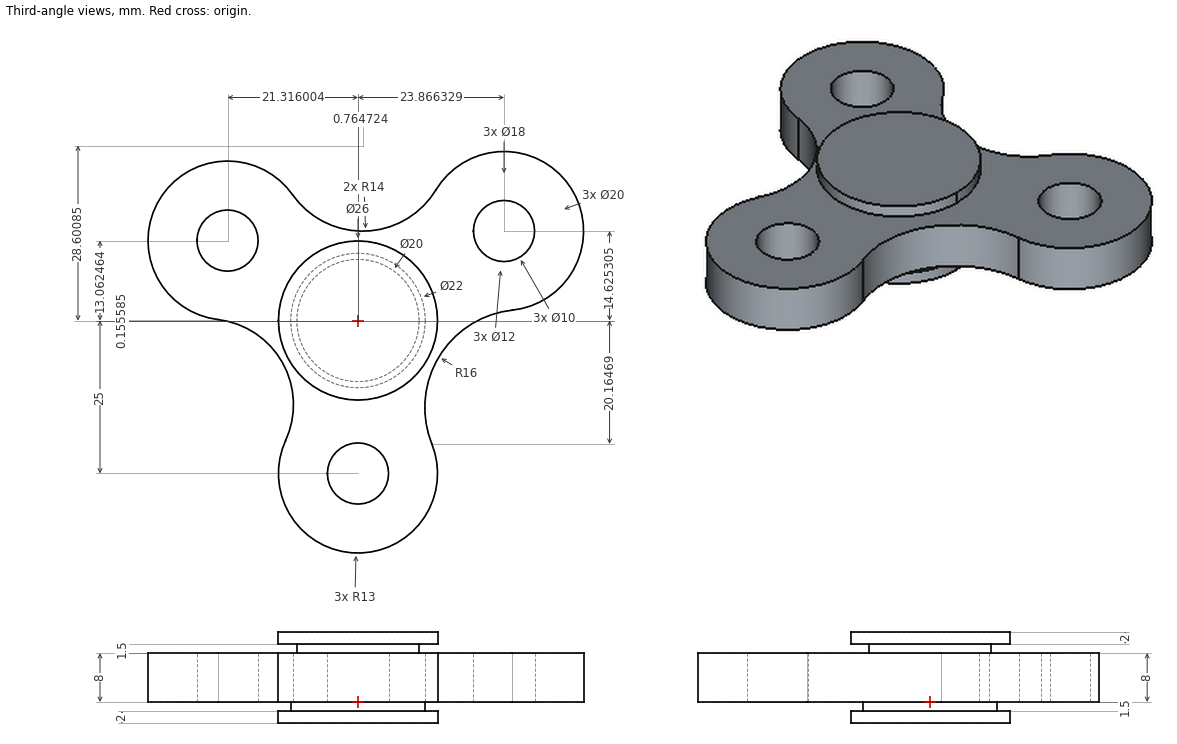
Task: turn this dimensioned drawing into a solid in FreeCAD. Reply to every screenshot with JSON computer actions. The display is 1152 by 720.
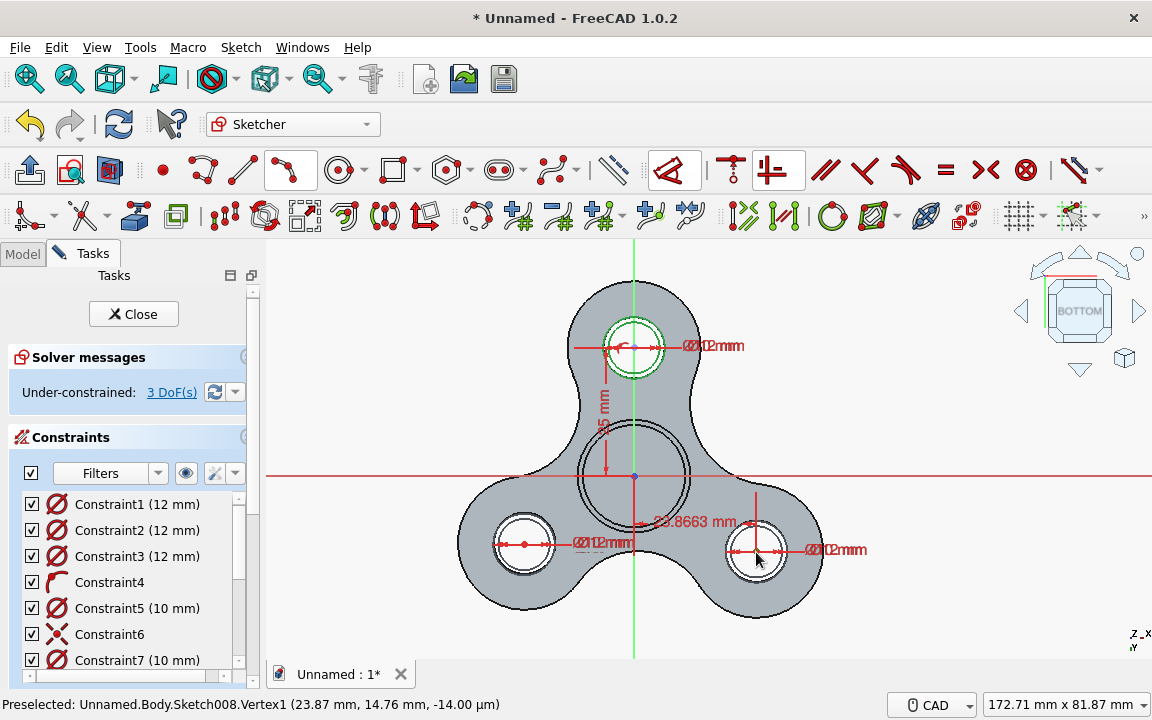
{"action": "left_click", "coordinate": [696, 170]}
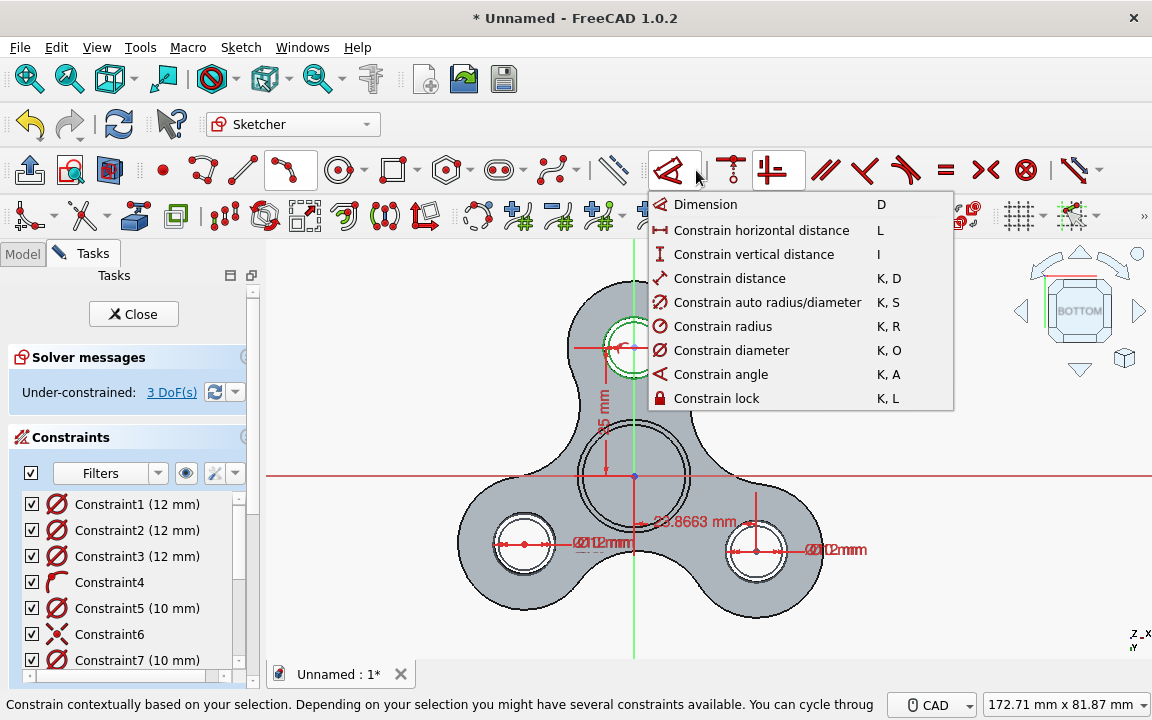
{"action": "left_click", "coordinate": [801, 254]}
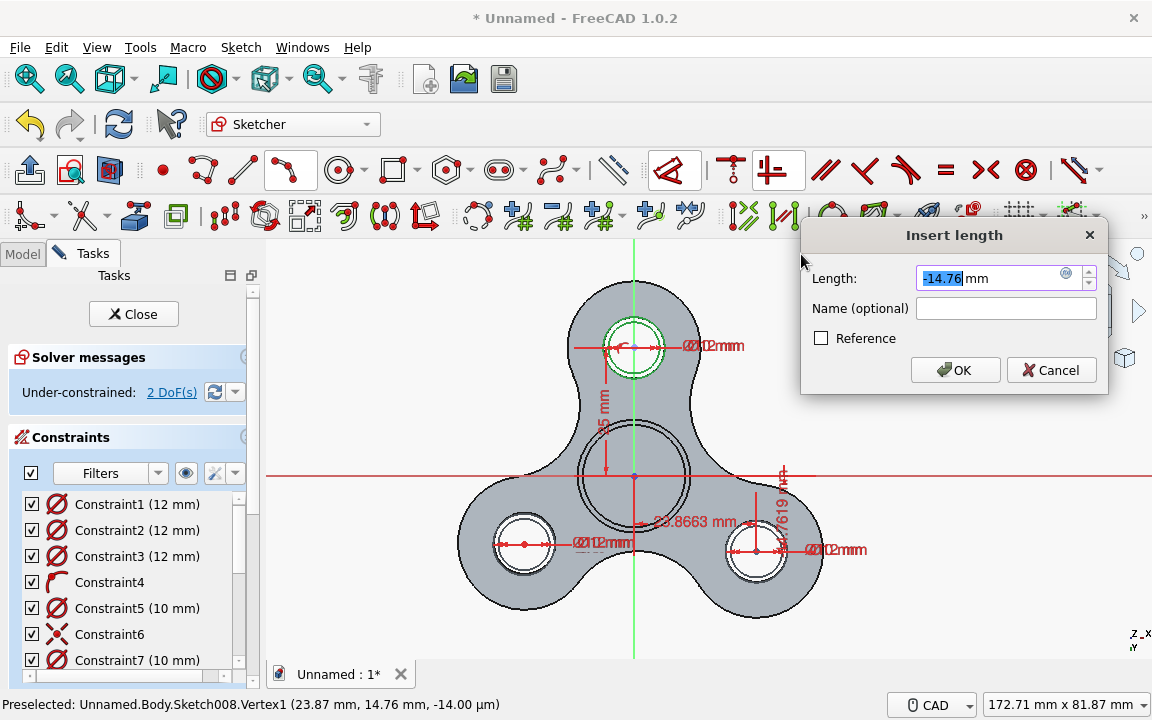
{"action": "type", "text": "-14.625305"}
{"action": "key", "text": "Return"}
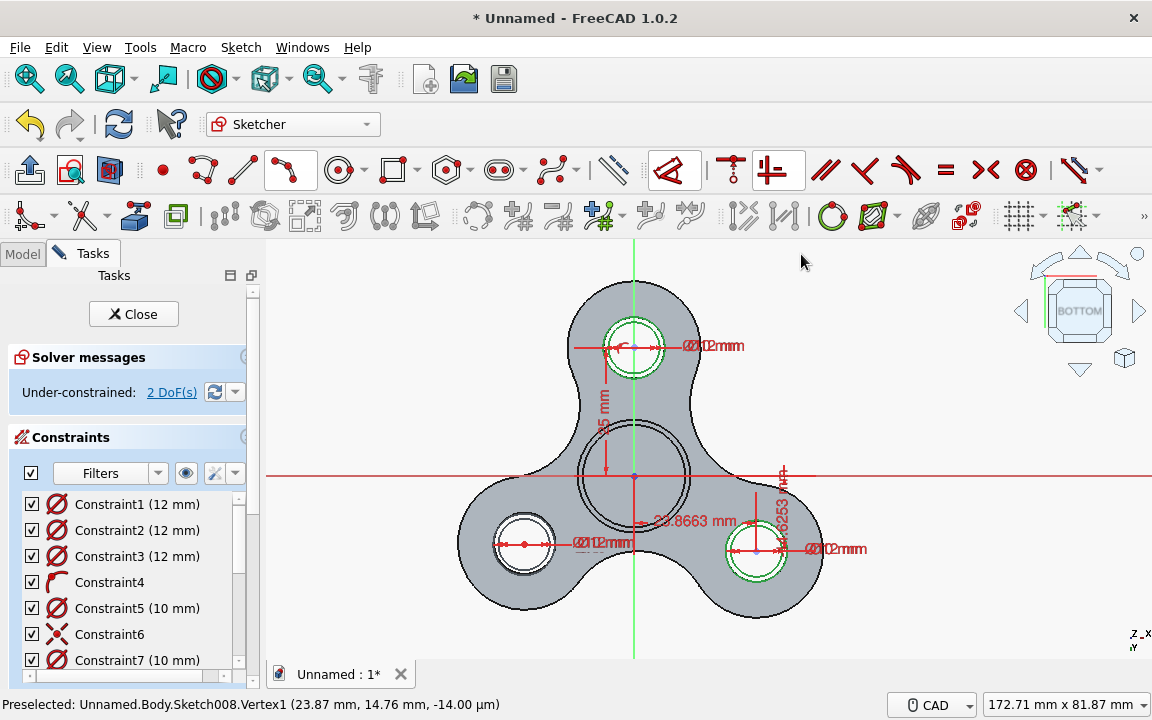
{"action": "left_click", "coordinate": [524, 545]}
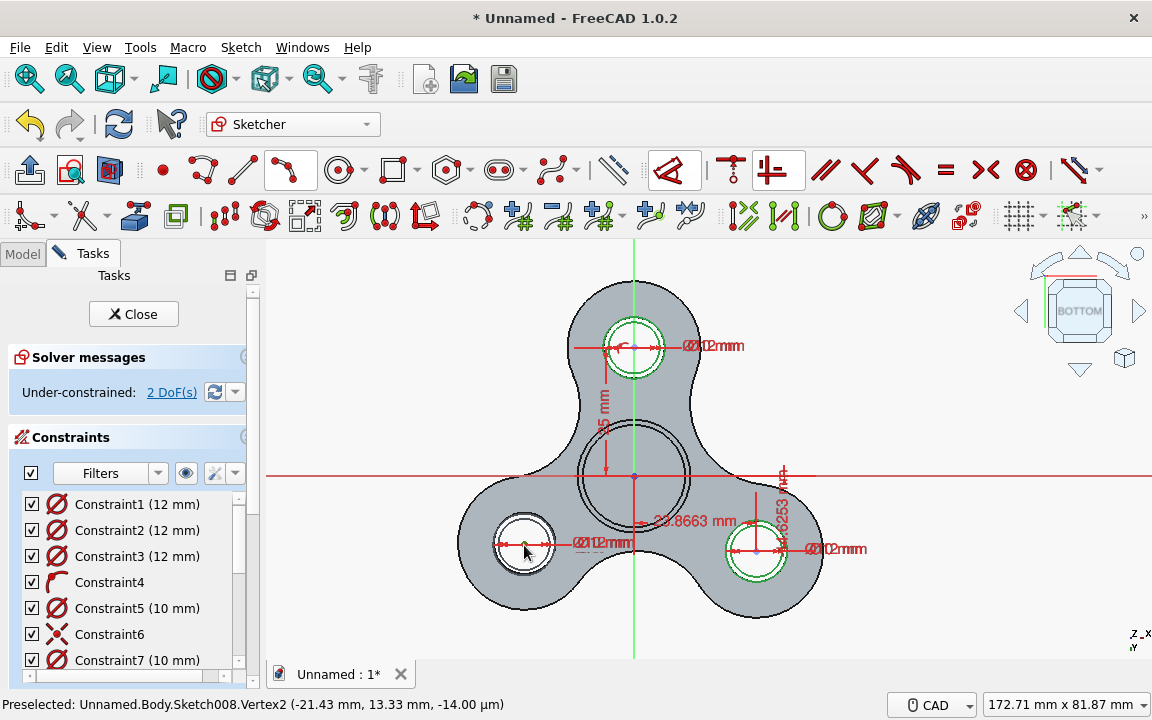
{"action": "left_click", "coordinate": [696, 170]}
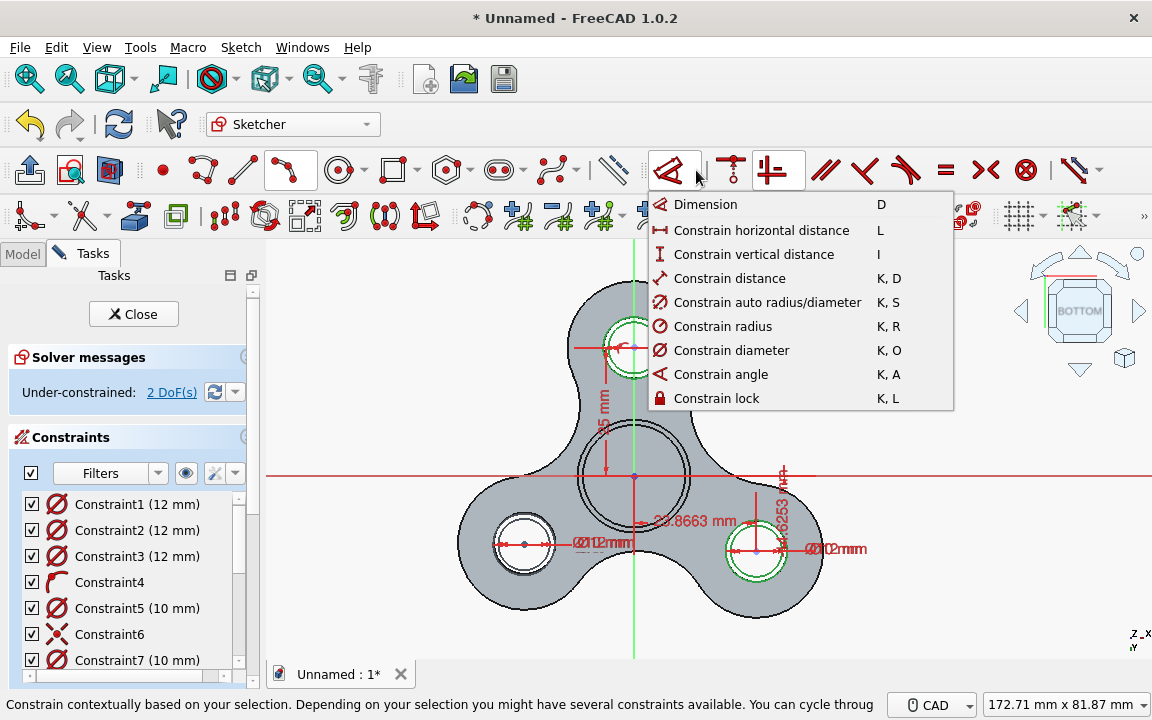
{"action": "left_click", "coordinate": [801, 230]}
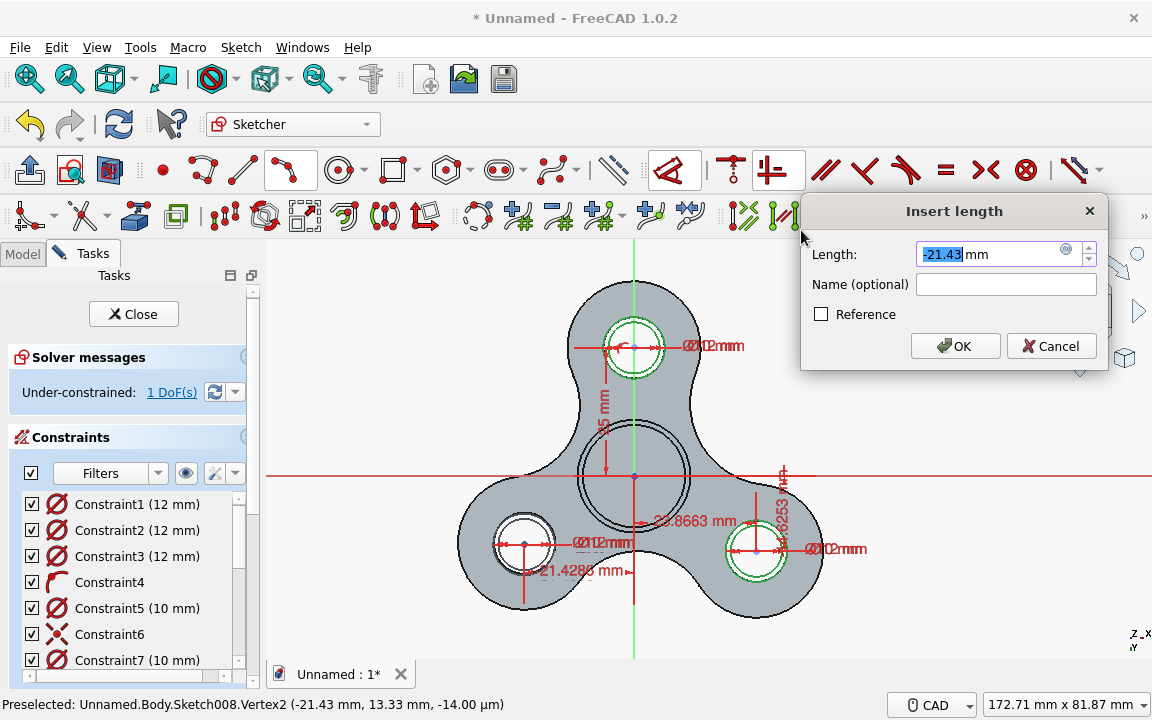
{"action": "type", "text": "-21.316004"}
{"action": "key", "text": "Return"}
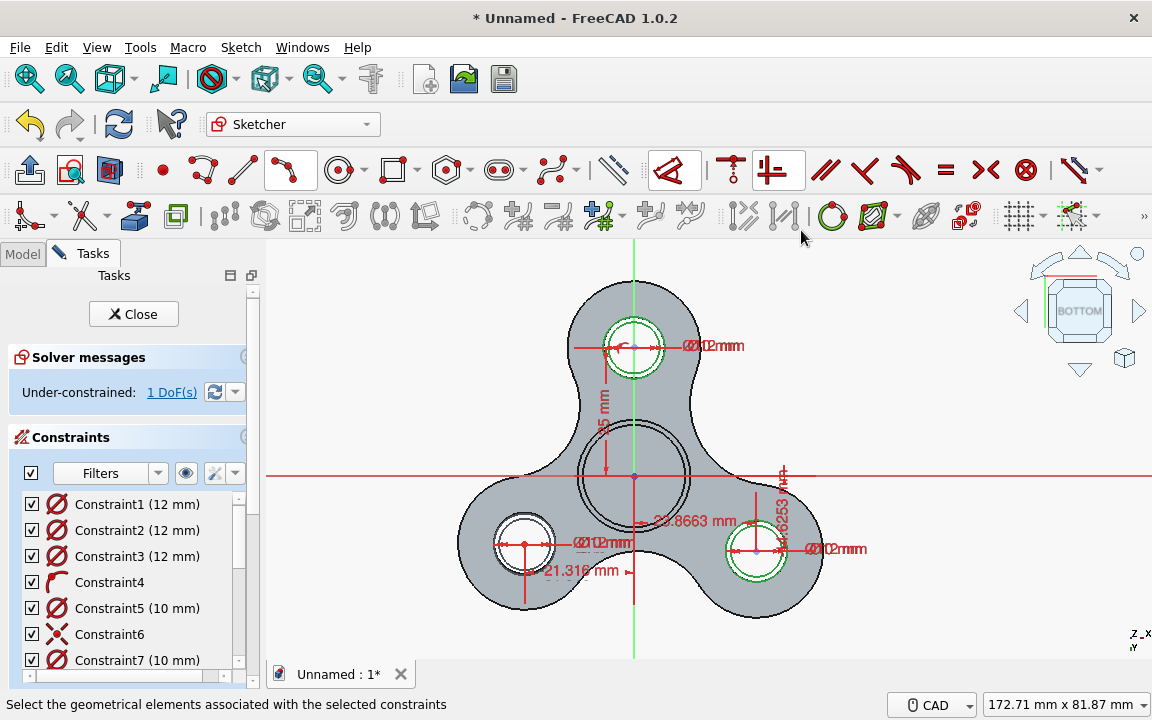
{"action": "left_click", "coordinate": [525, 545]}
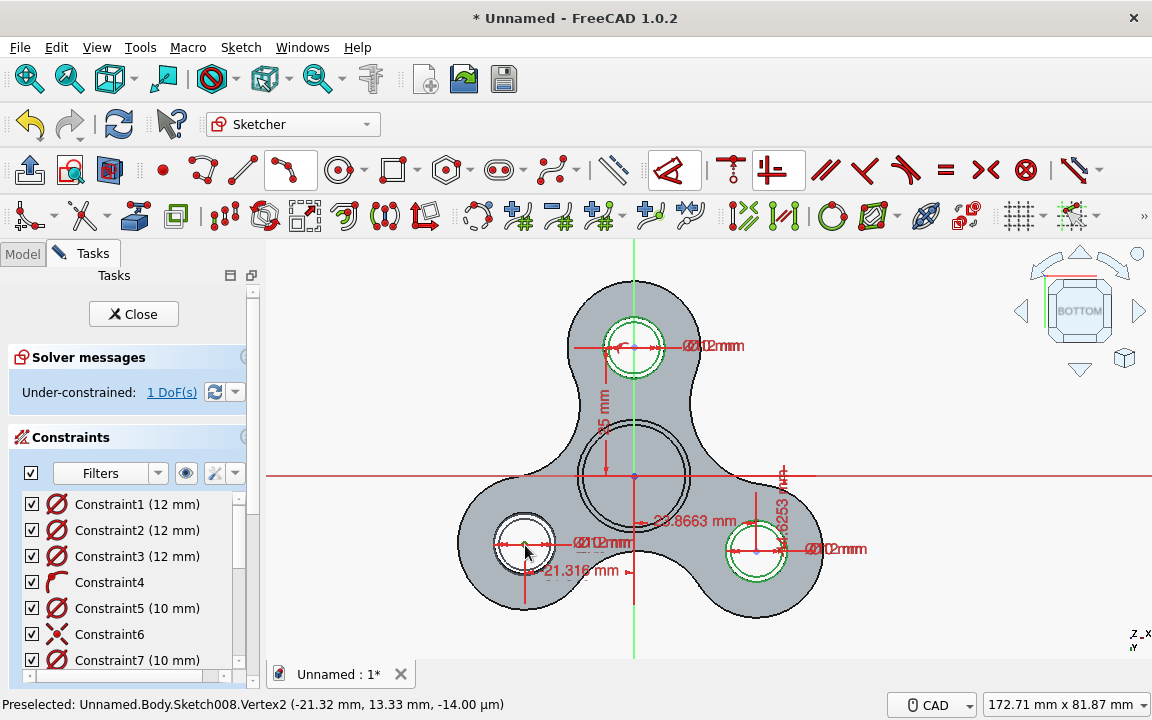
{"action": "key", "text": "i"}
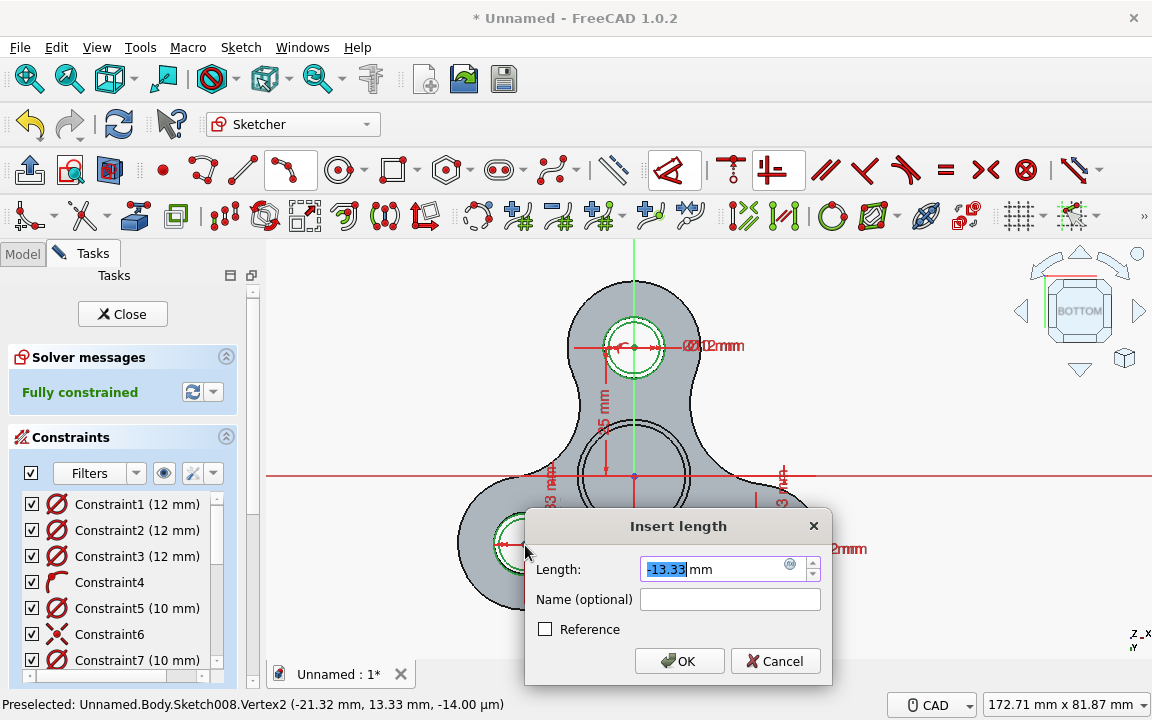
{"action": "type", "text": "-13.062464"}
{"action": "key", "text": "Return"}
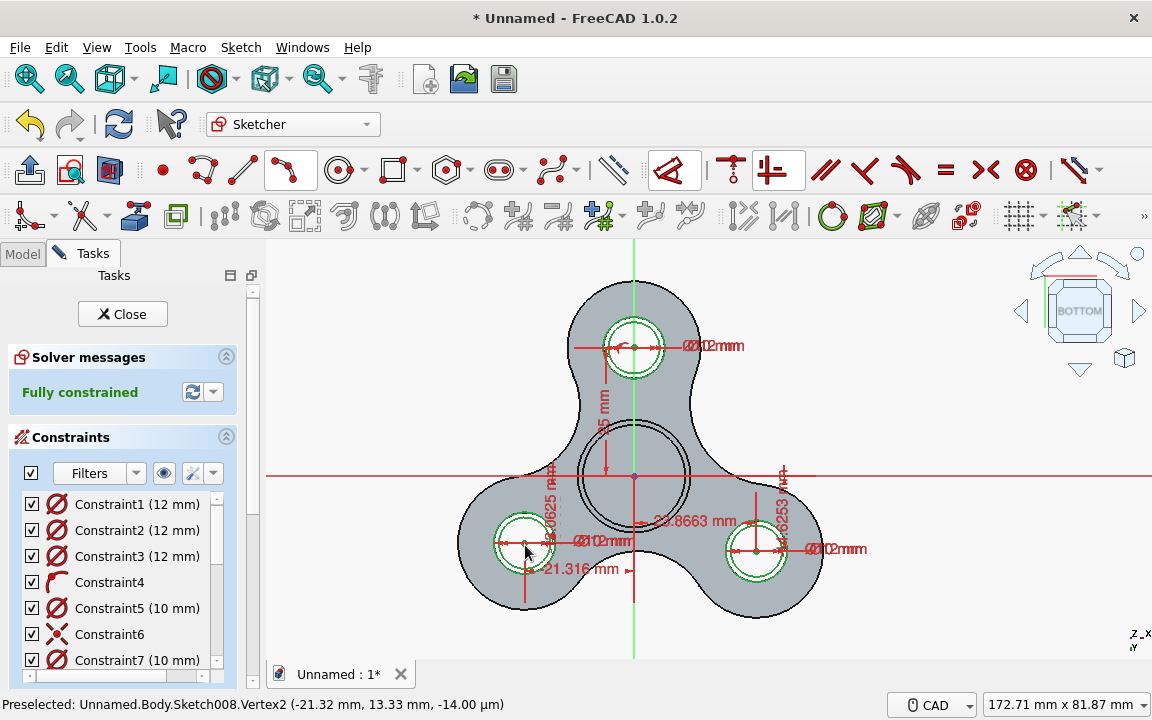
{"action": "left_click", "coordinate": [123, 314]}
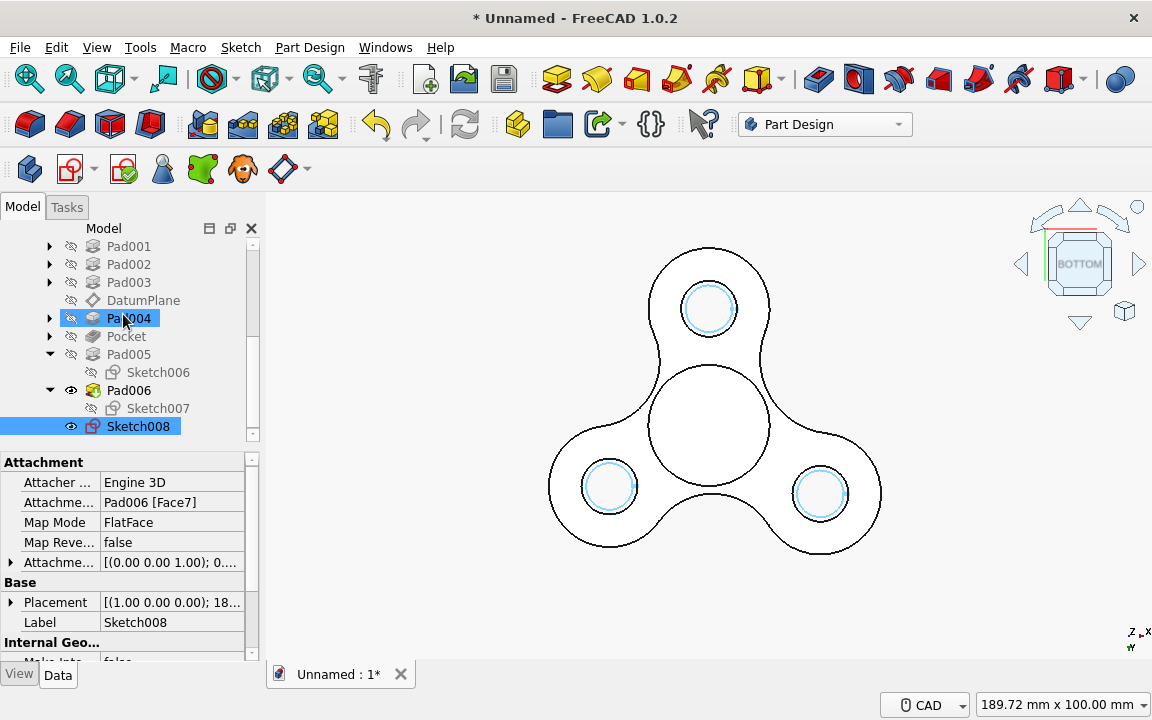
{"action": "left_click", "coordinate": [558, 80]}